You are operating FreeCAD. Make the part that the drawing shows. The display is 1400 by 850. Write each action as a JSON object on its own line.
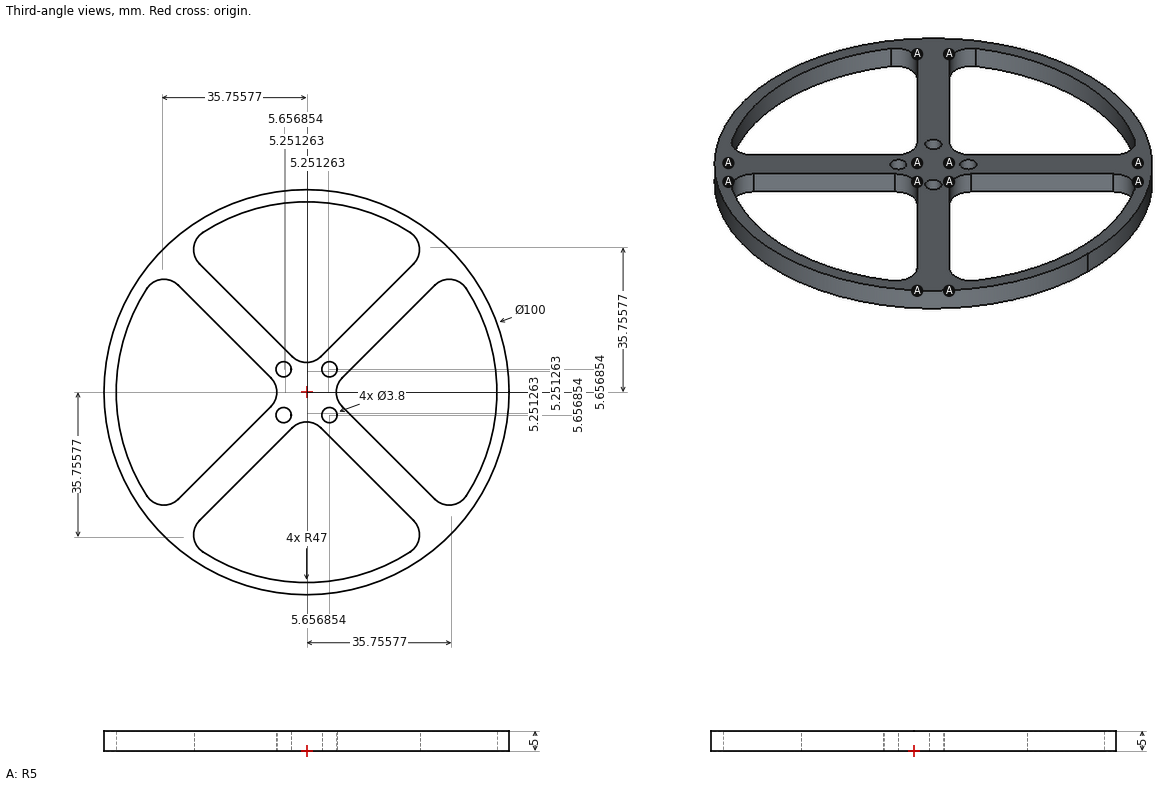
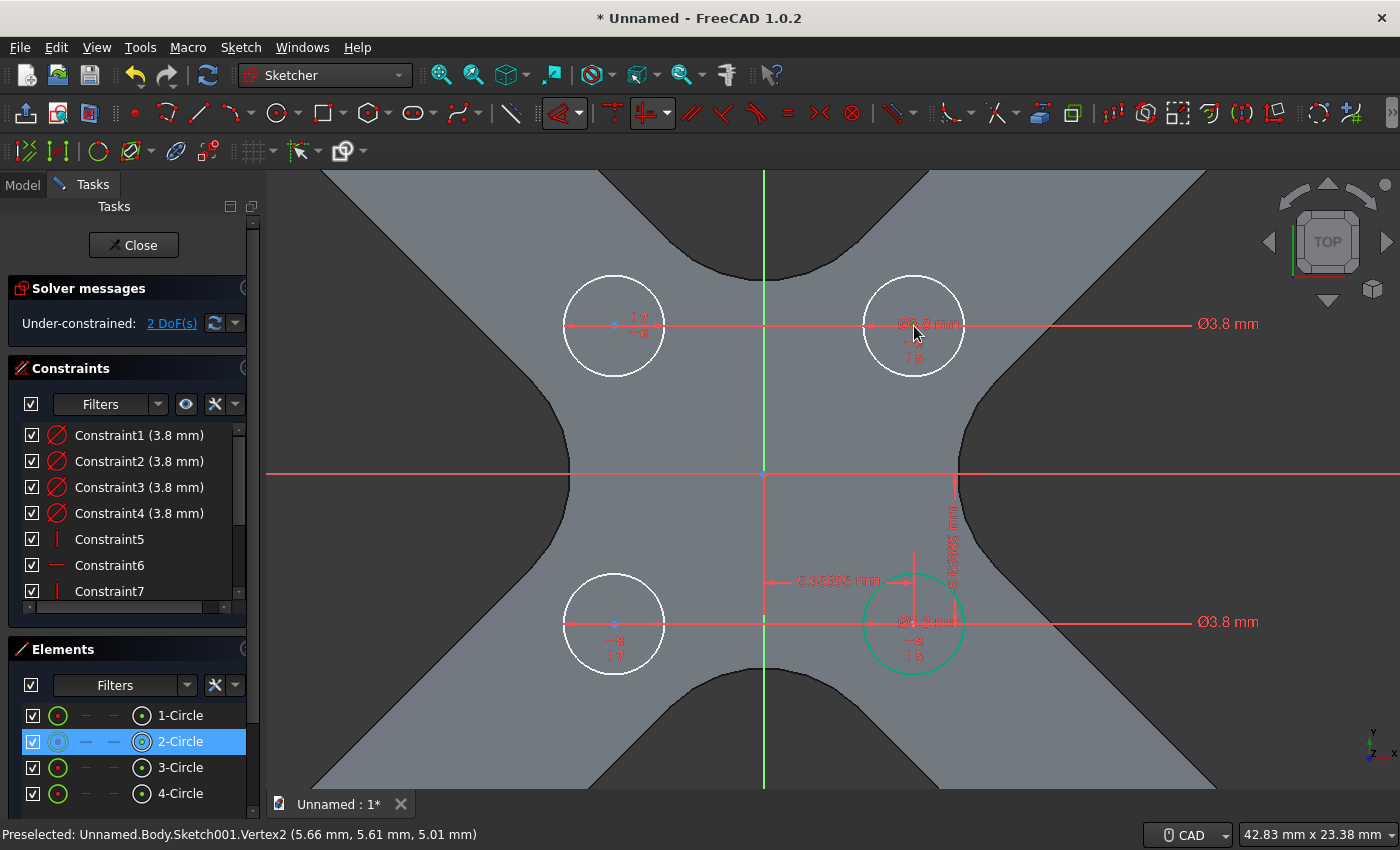
{"action": "left_click", "coordinate": [582, 114]}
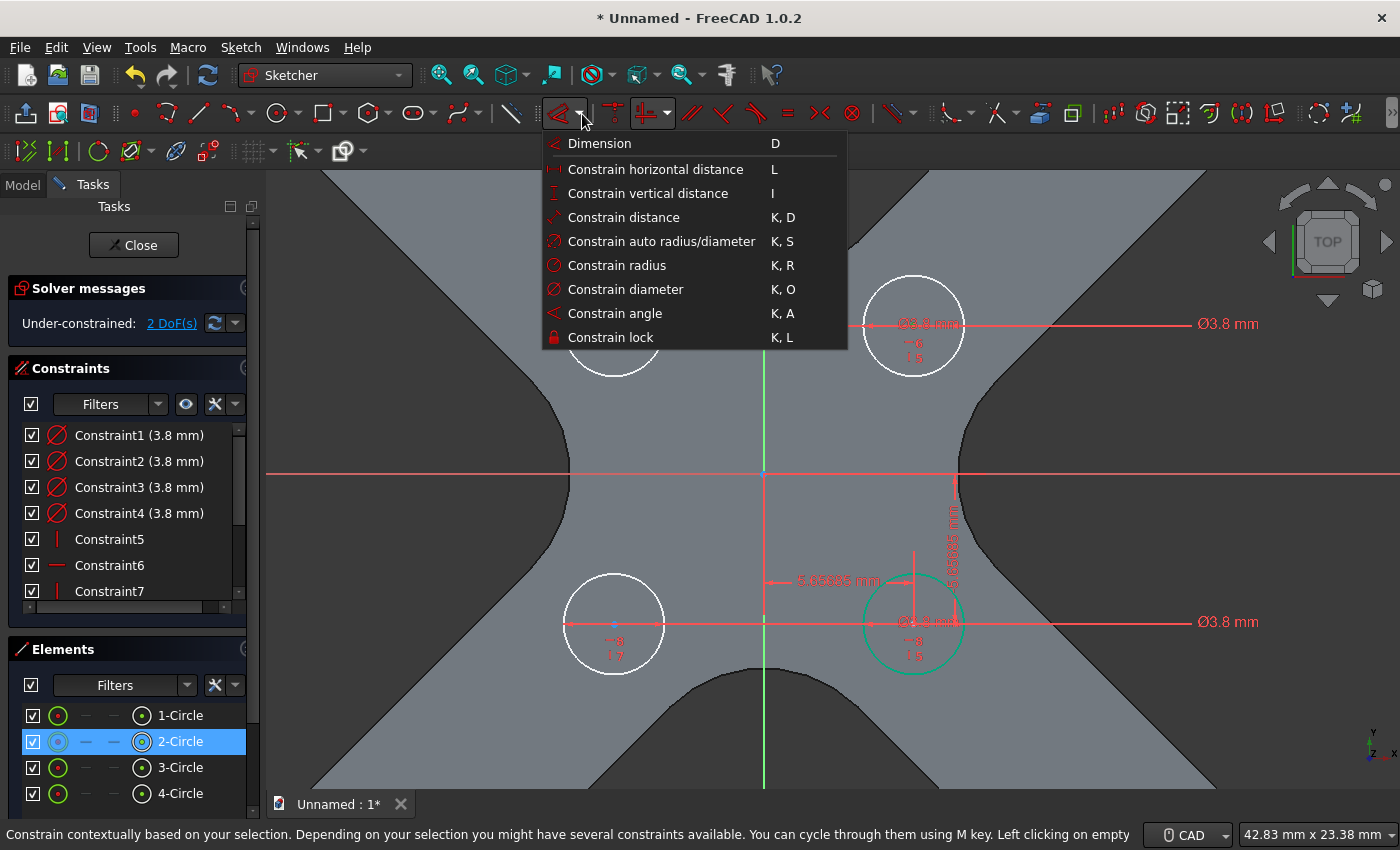
{"action": "left_click", "coordinate": [695, 193]}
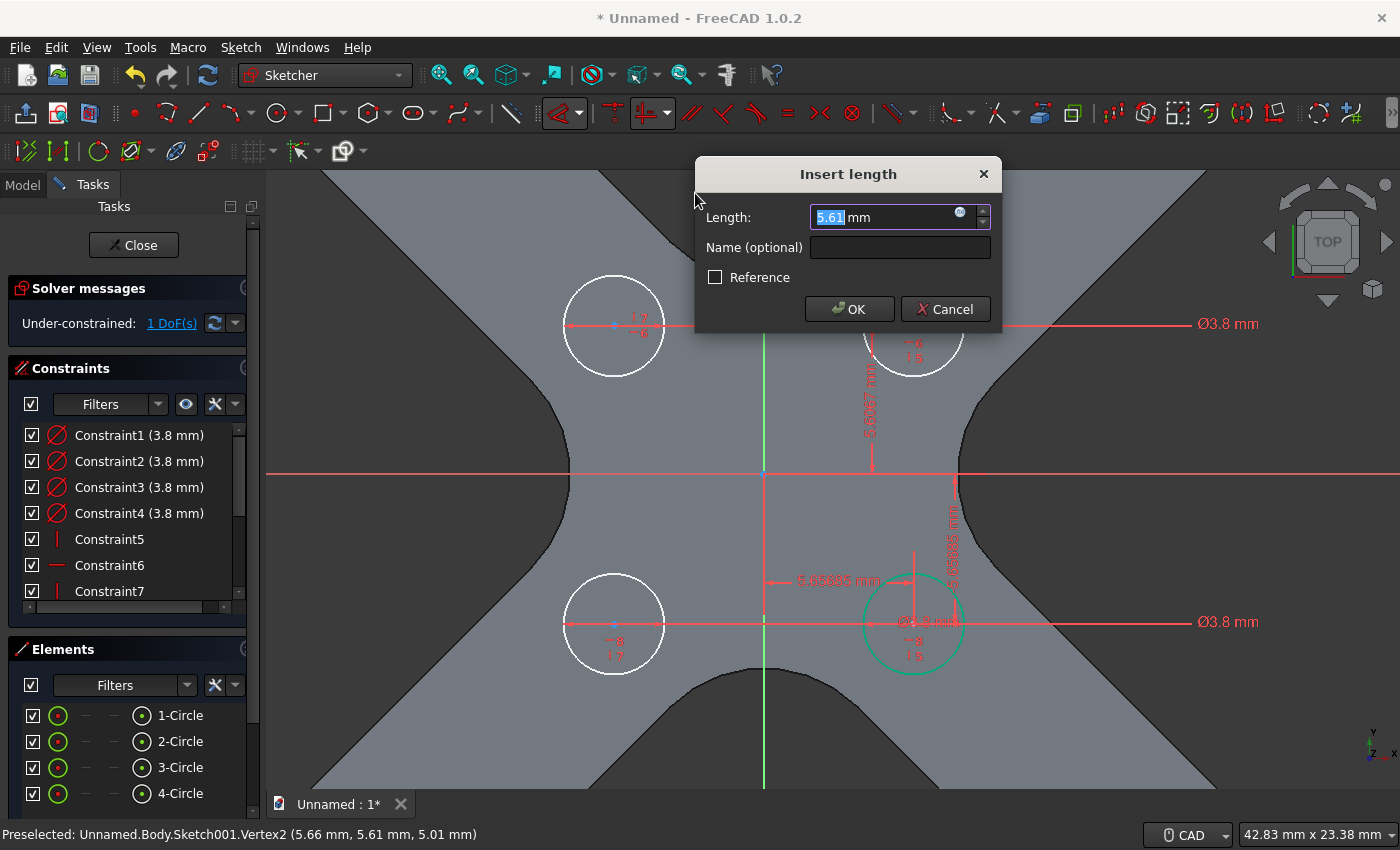
{"action": "type", "text": "5.656854"}
{"action": "key", "text": "Return"}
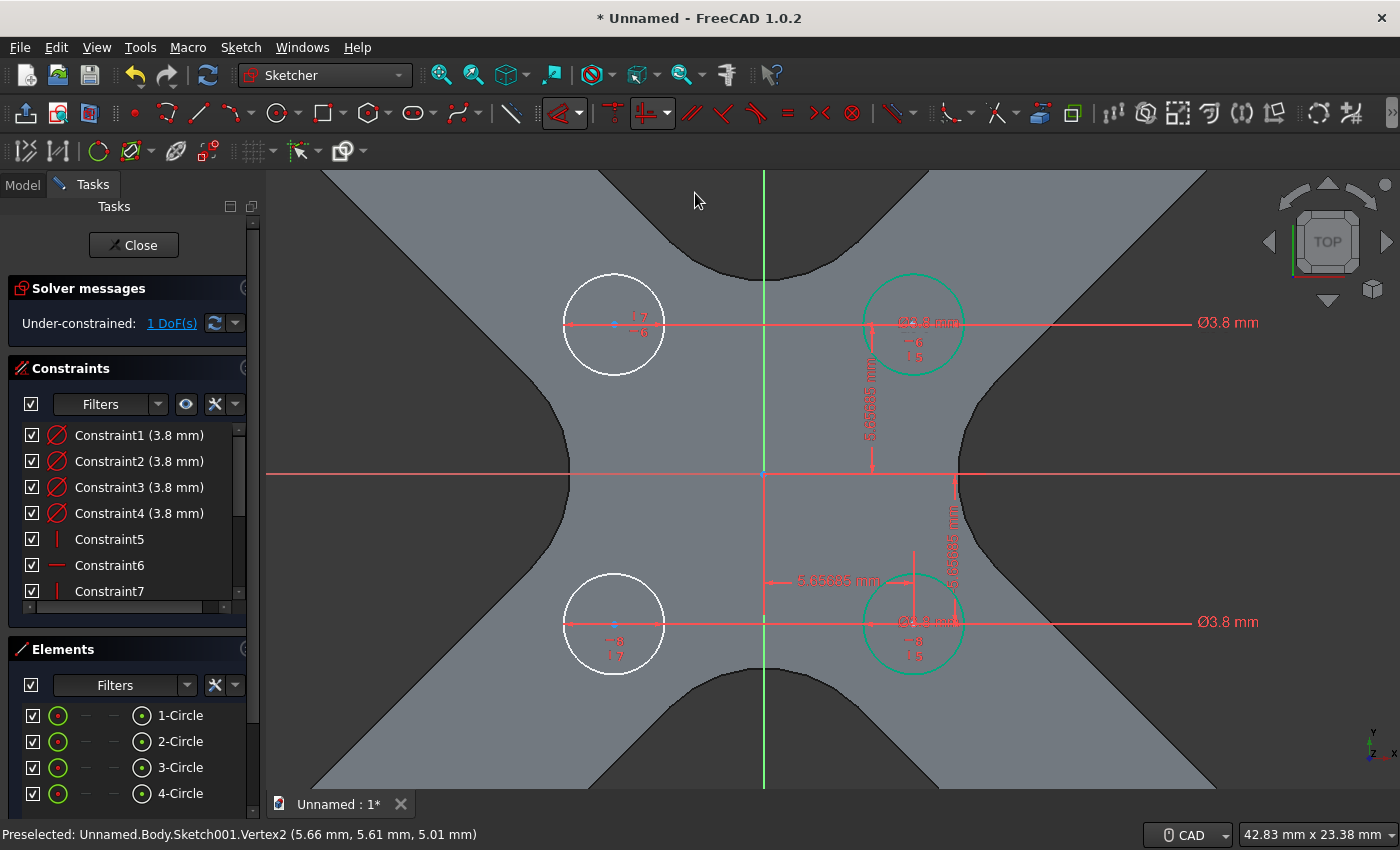
{"action": "left_click", "coordinate": [614, 325]}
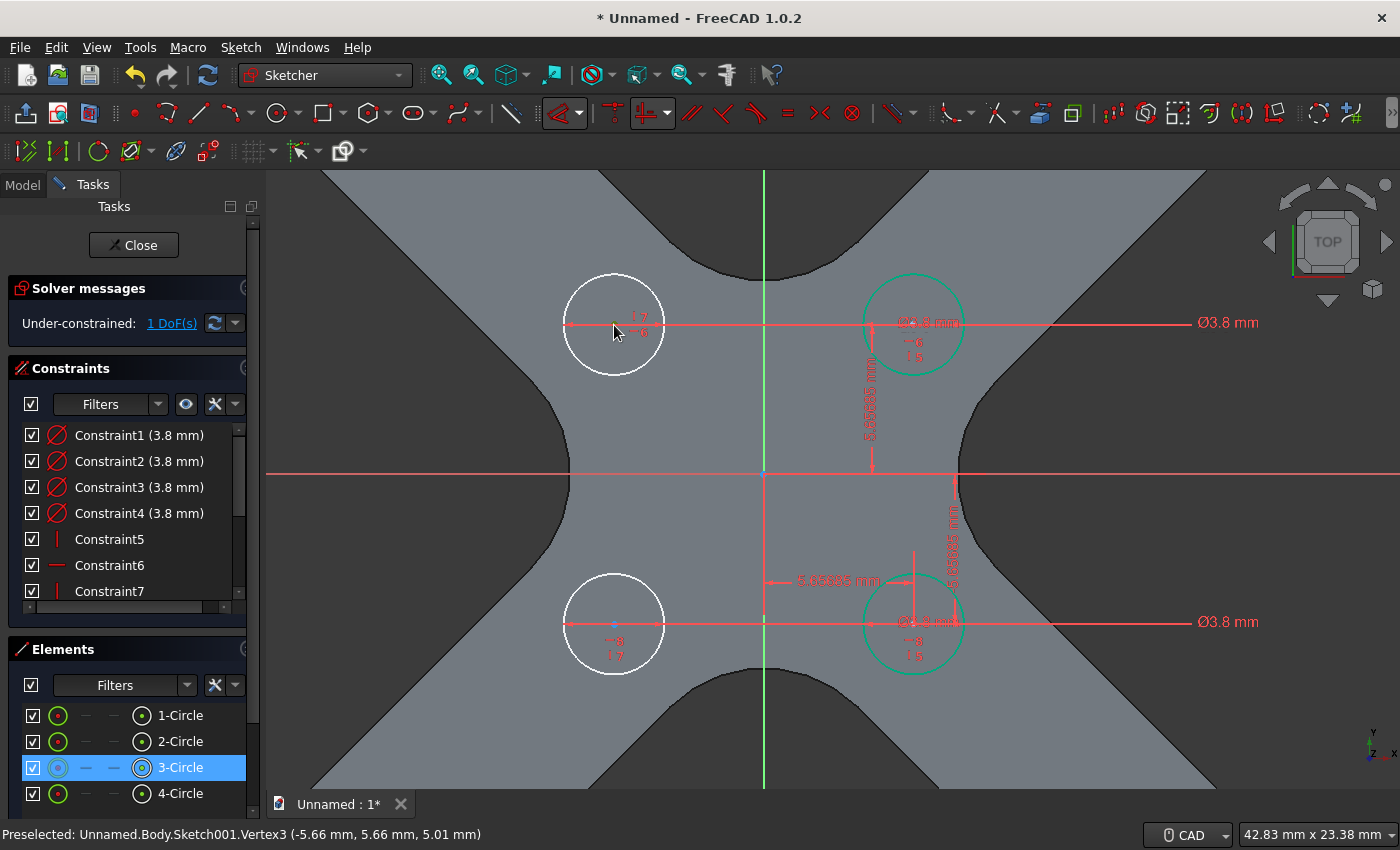
{"action": "left_click", "coordinate": [582, 114]}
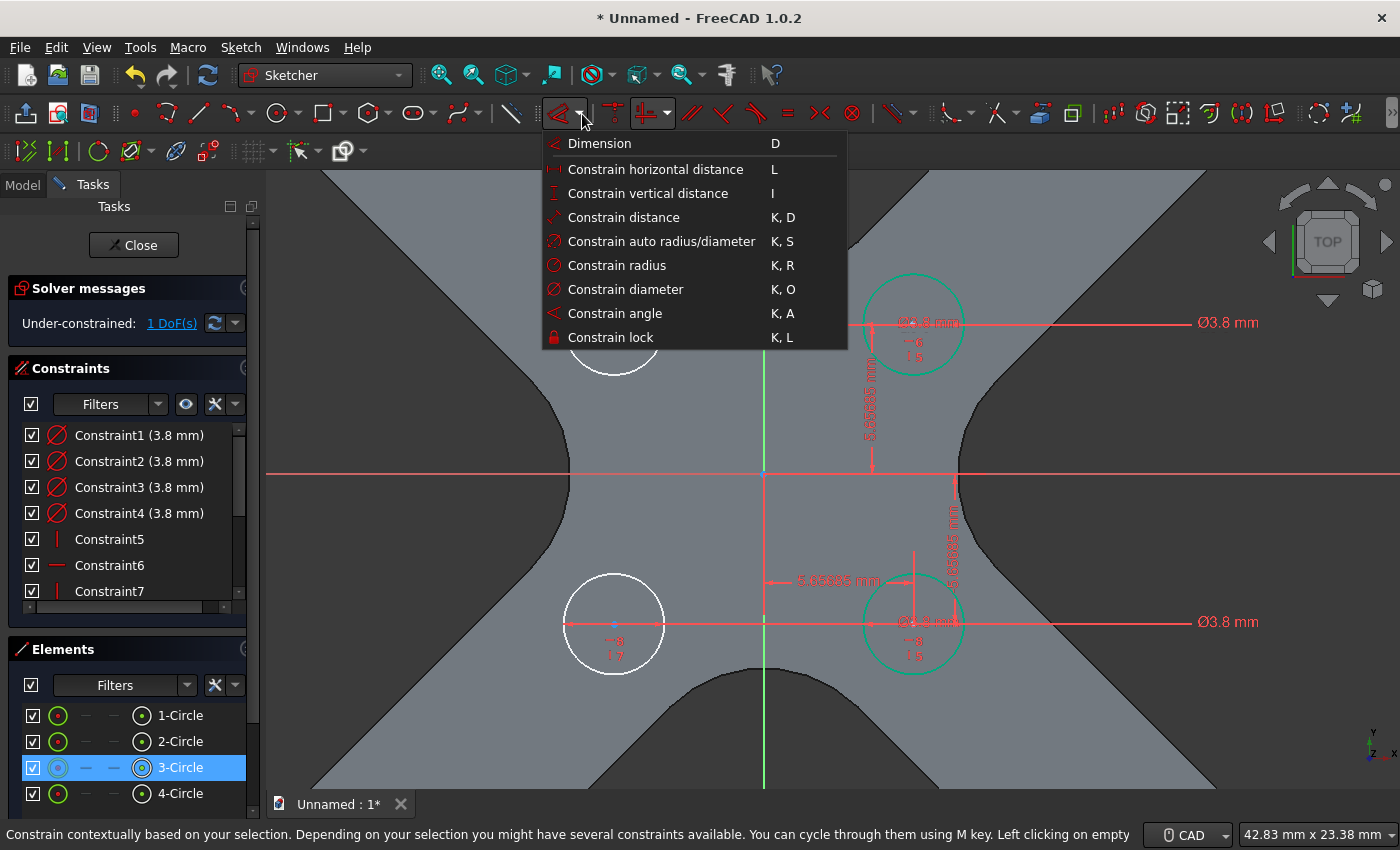
{"action": "left_click", "coordinate": [695, 169]}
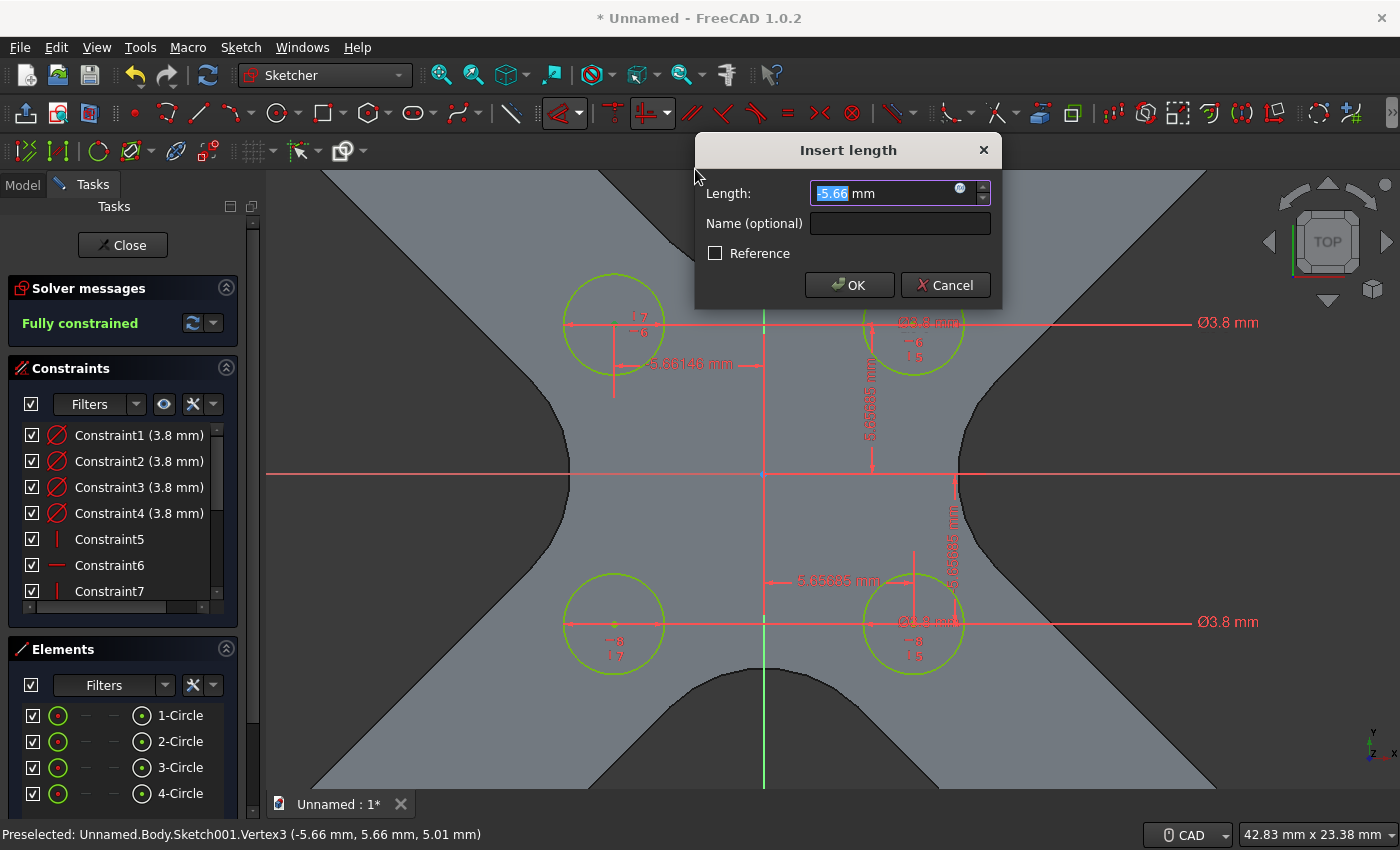
{"action": "type", "text": "-5.656854"}
{"action": "key", "text": "Return"}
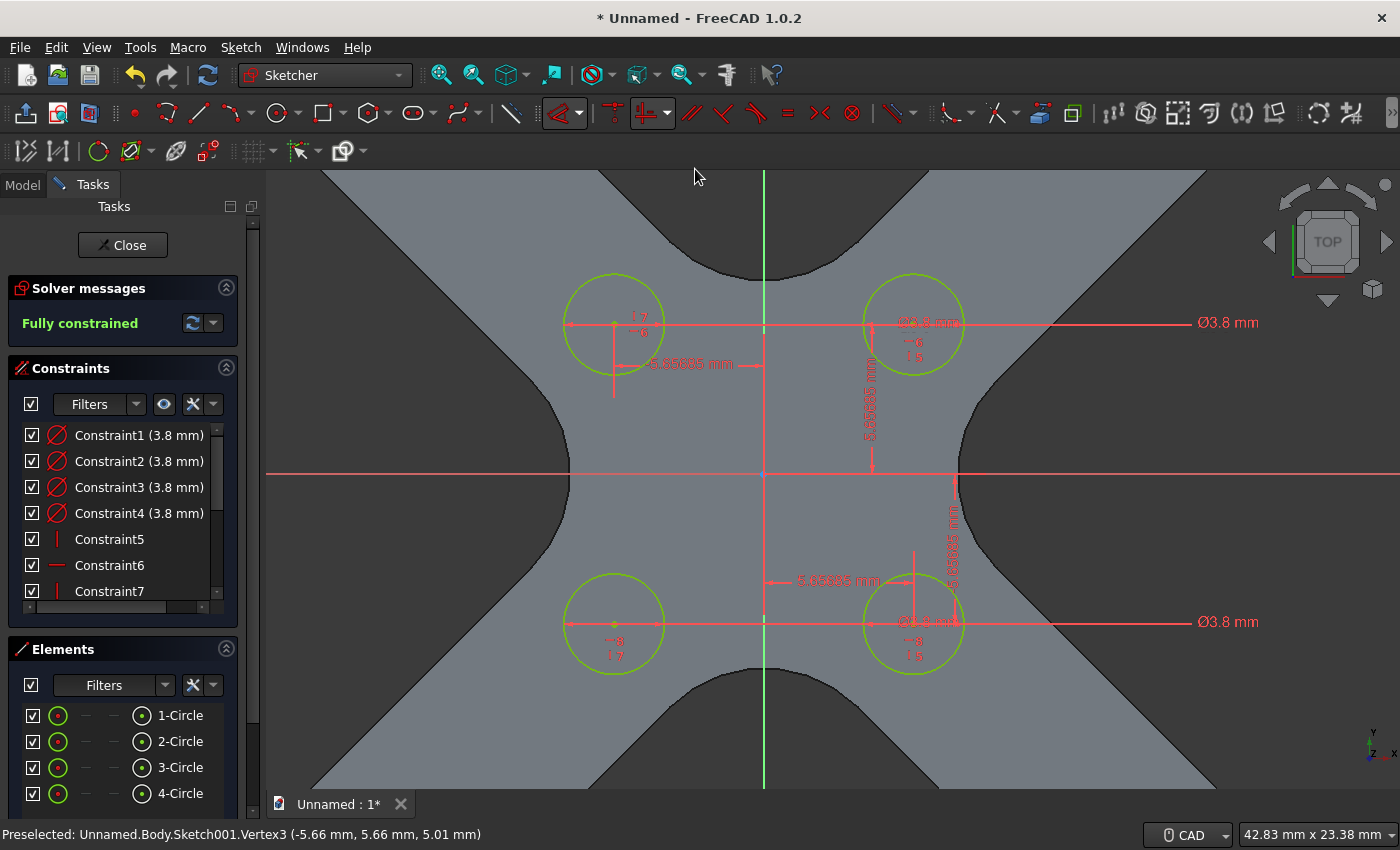
{"action": "left_click", "coordinate": [123, 245]}